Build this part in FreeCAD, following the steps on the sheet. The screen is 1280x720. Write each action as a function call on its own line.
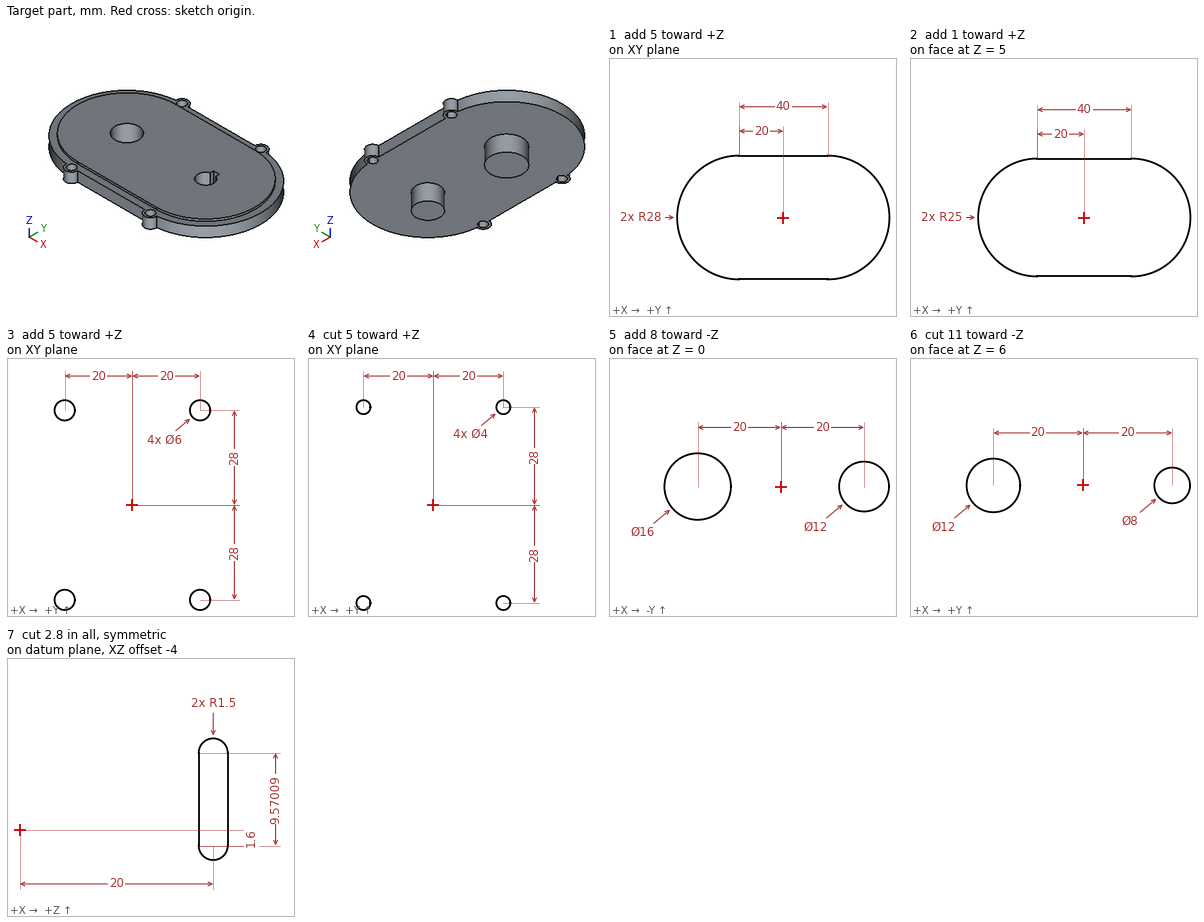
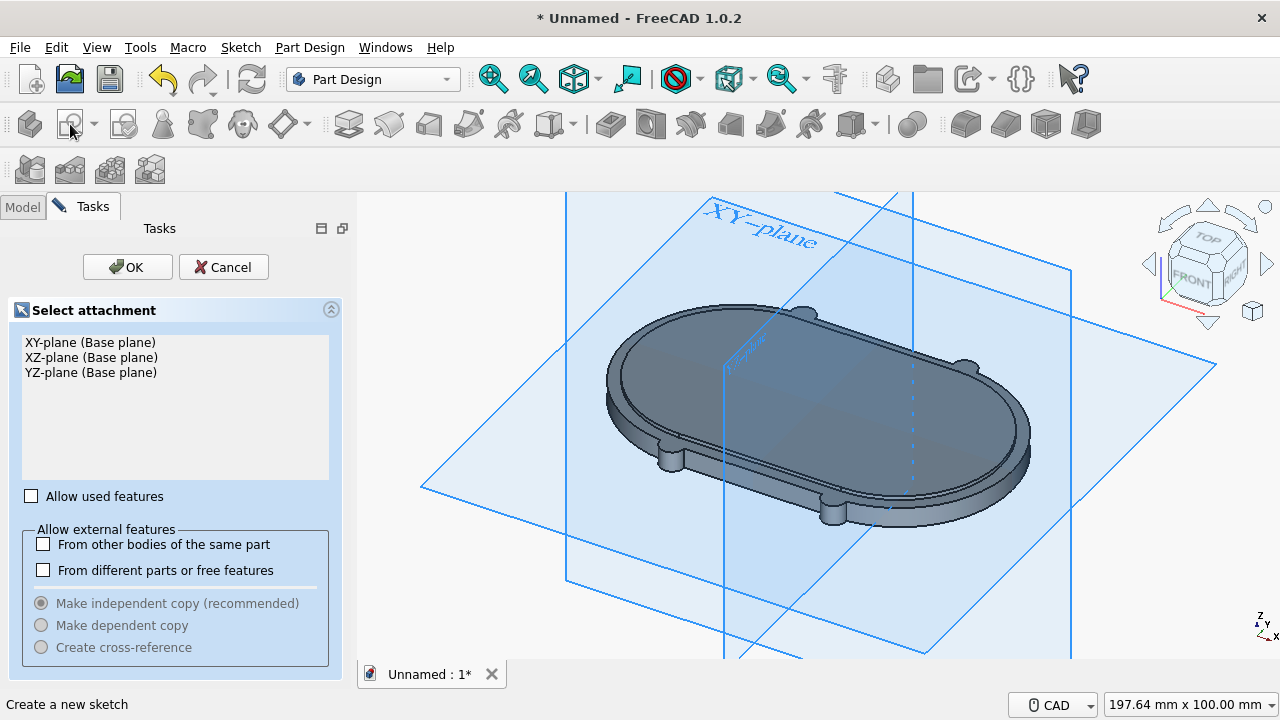
click(82, 342)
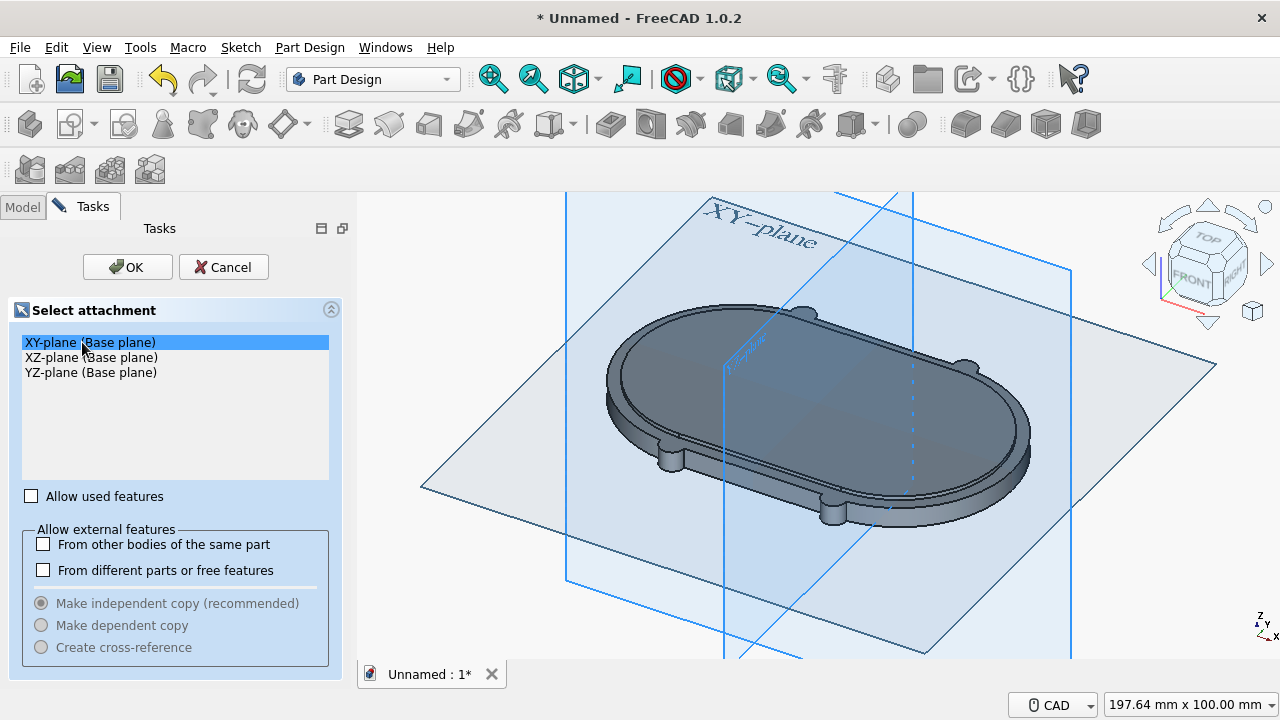
click(128, 267)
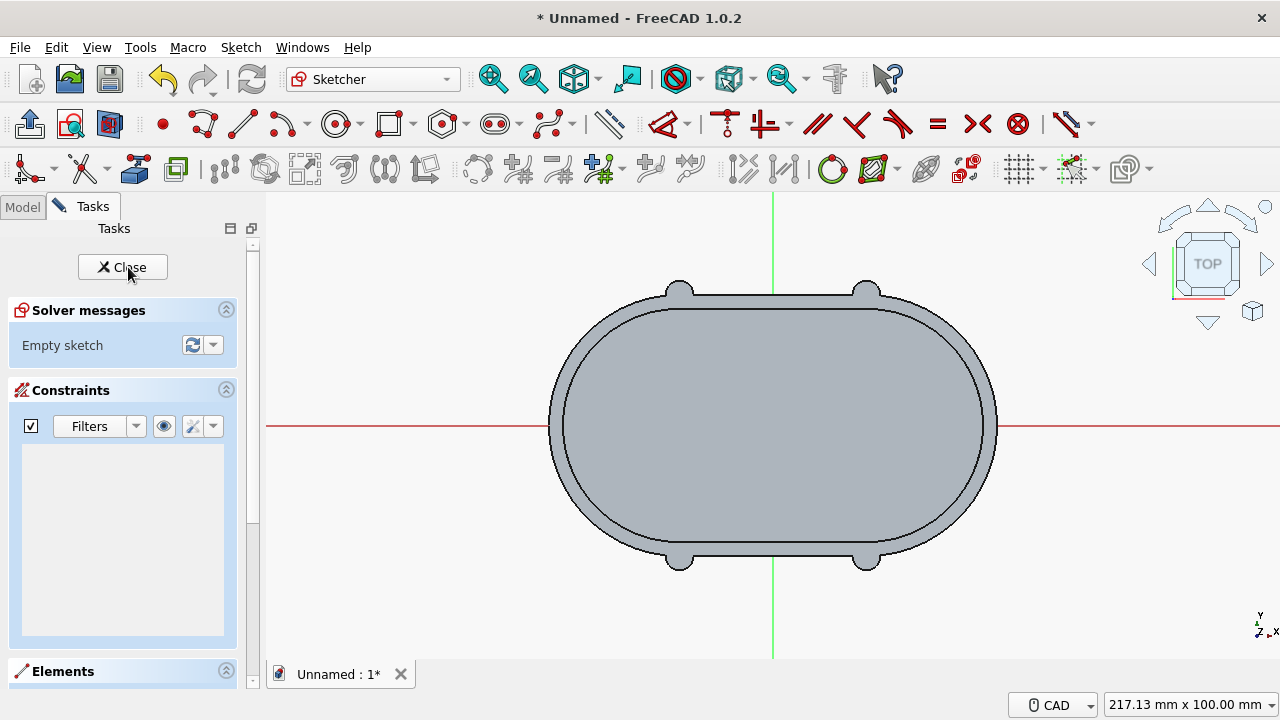
key(q)
key(s)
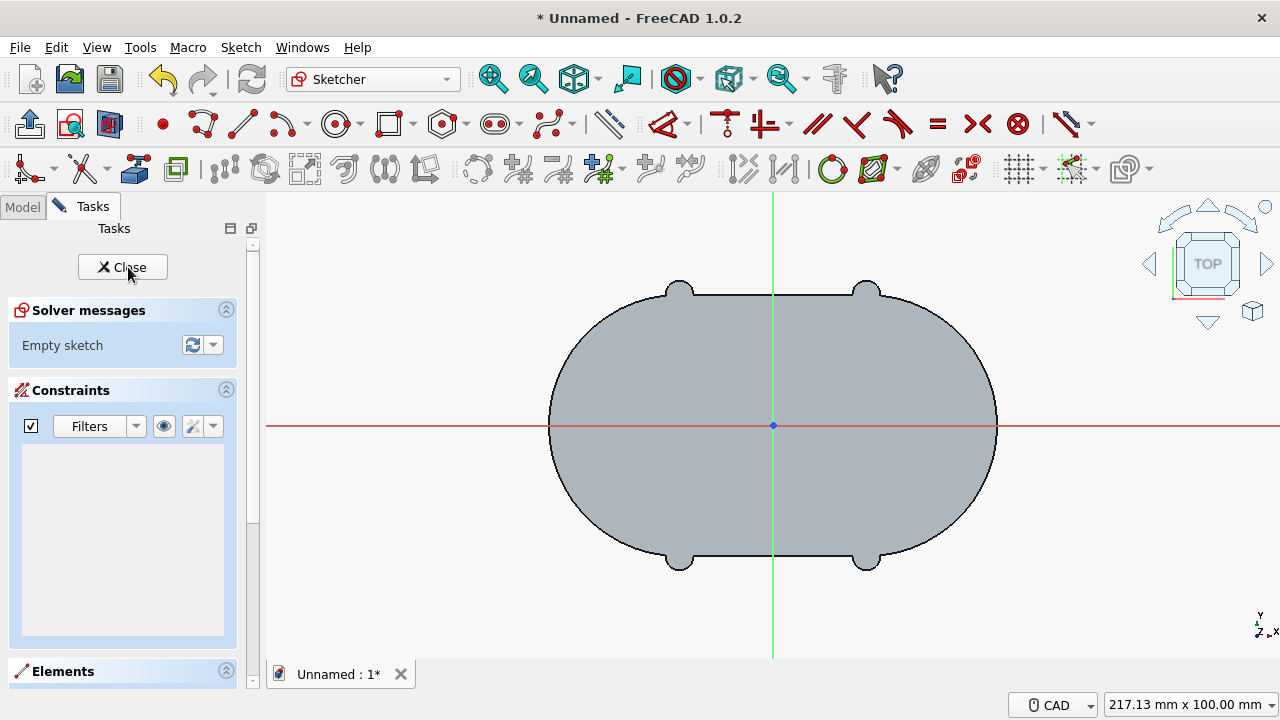
click(336, 124)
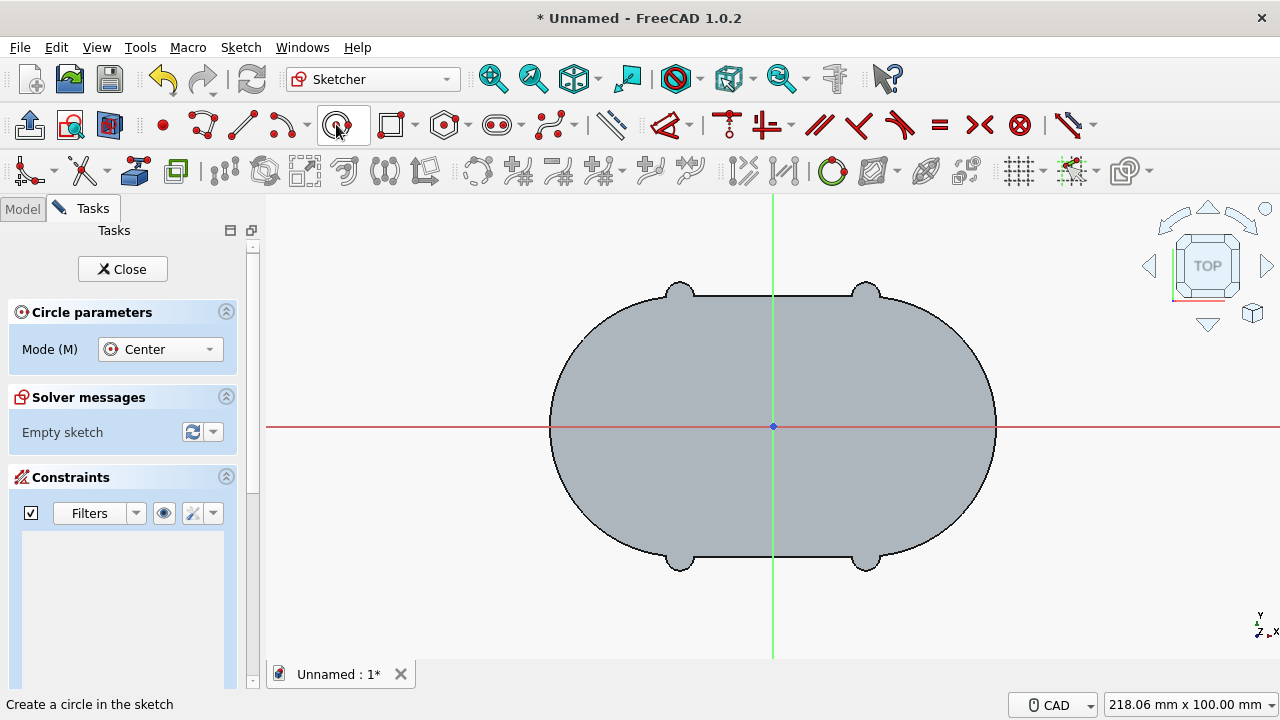
scroll(866, 296, up, 5)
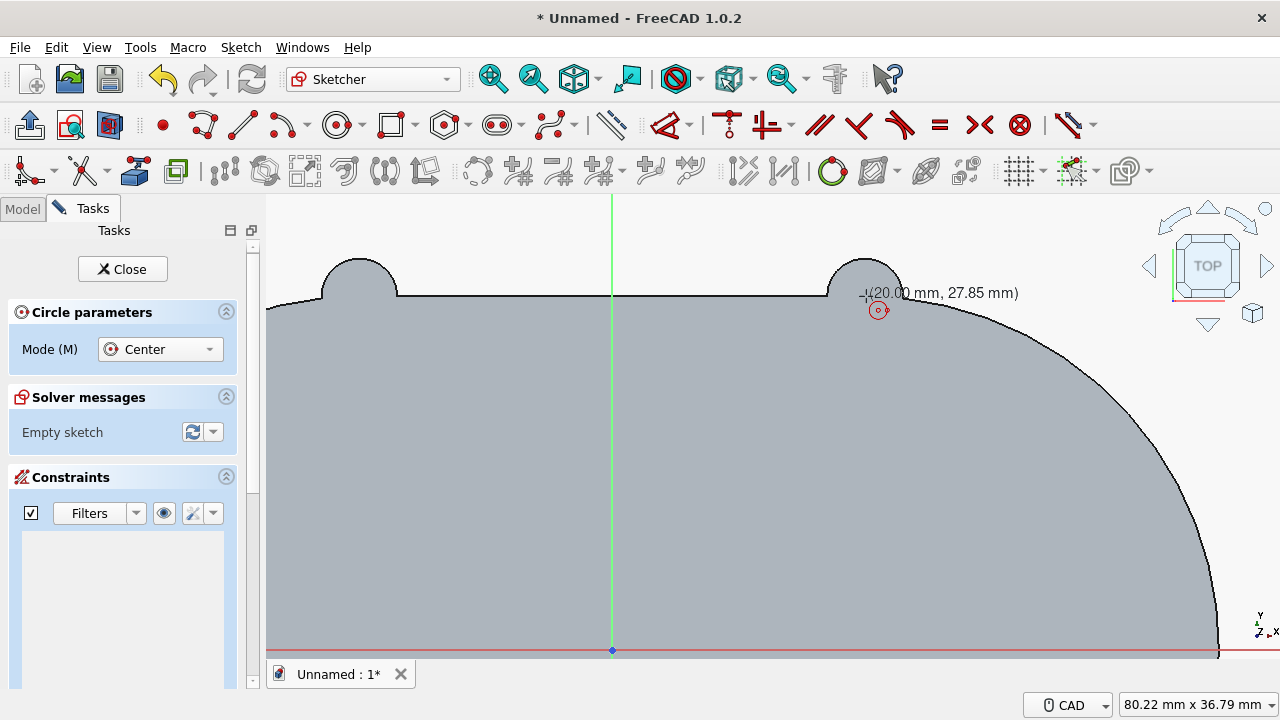
click(865, 296)
click(883, 279)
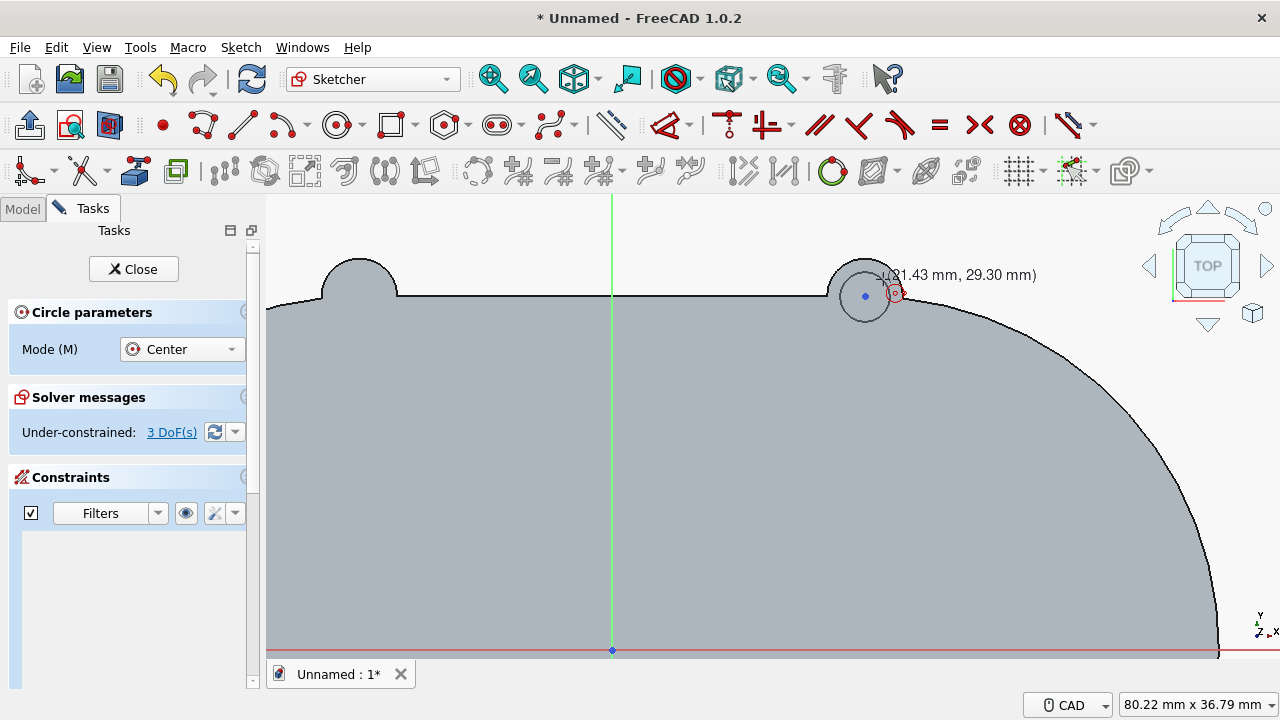
click(359, 296)
click(377, 279)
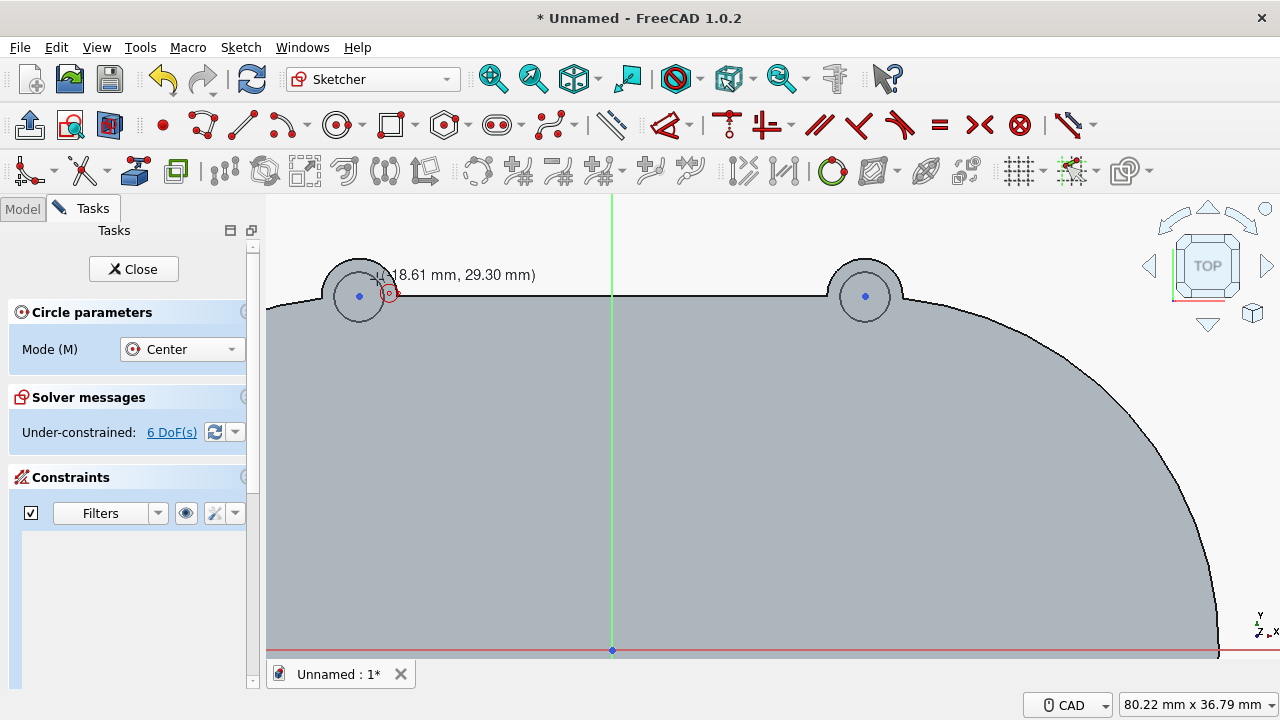
scroll(758, 296, down, 5)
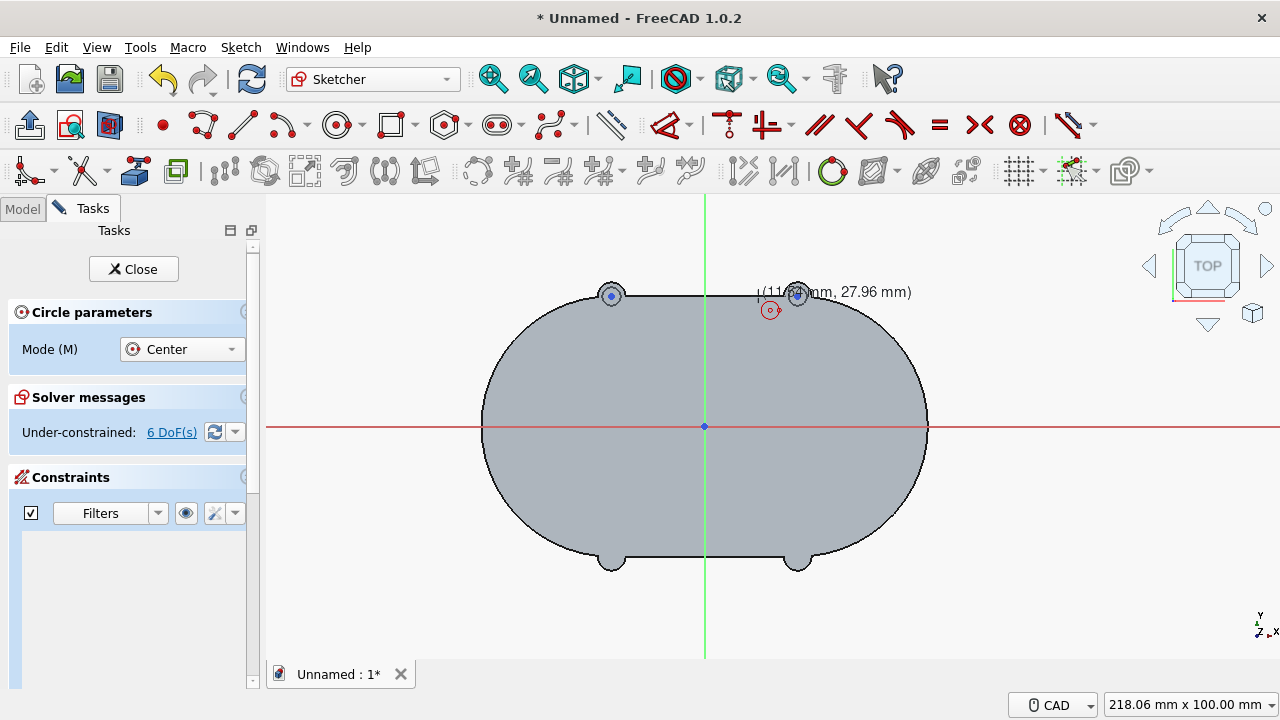
scroll(798, 557, up, 5)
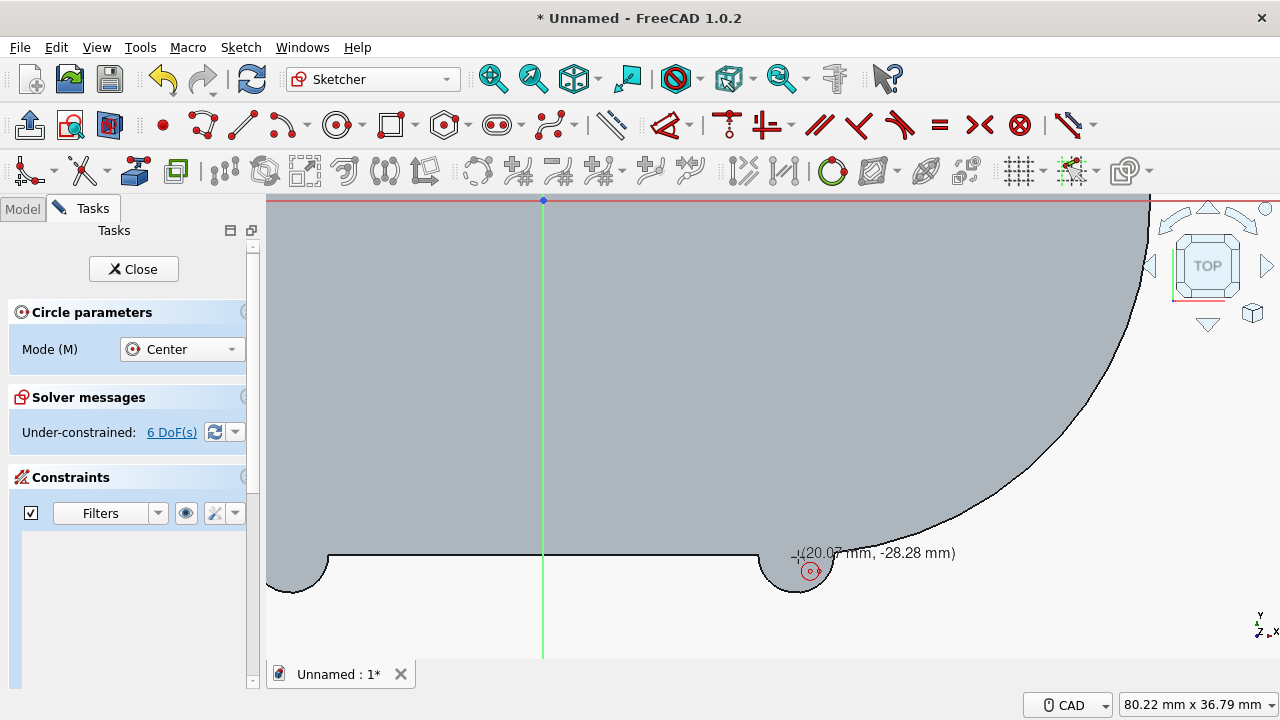
click(796, 555)
click(814, 537)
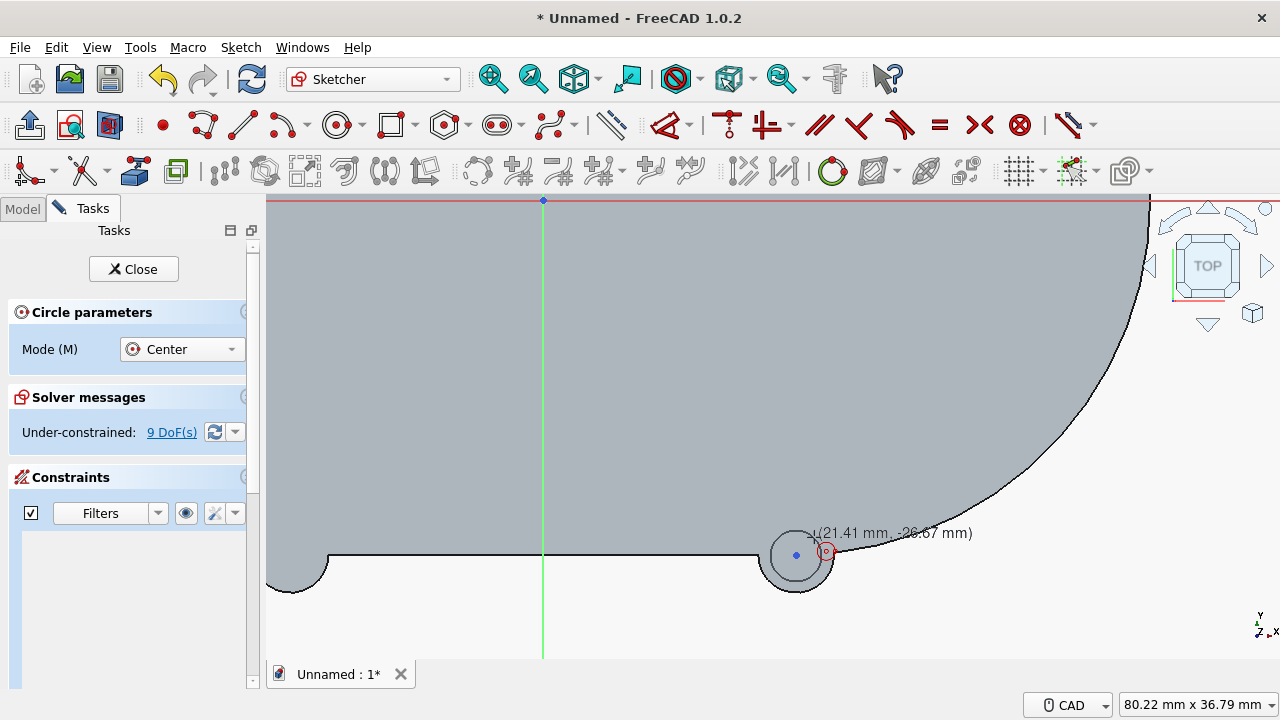
scroll(798, 558, down, 5)